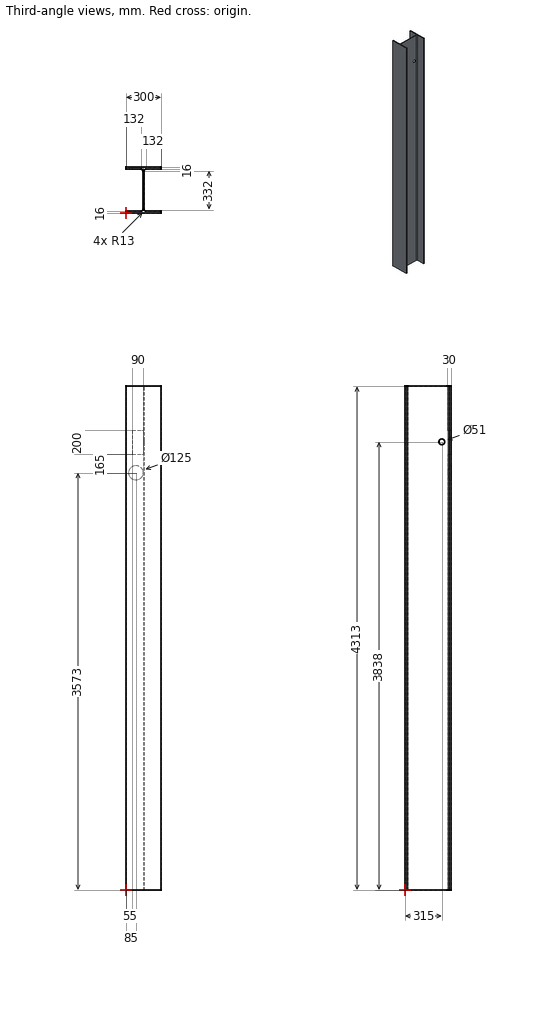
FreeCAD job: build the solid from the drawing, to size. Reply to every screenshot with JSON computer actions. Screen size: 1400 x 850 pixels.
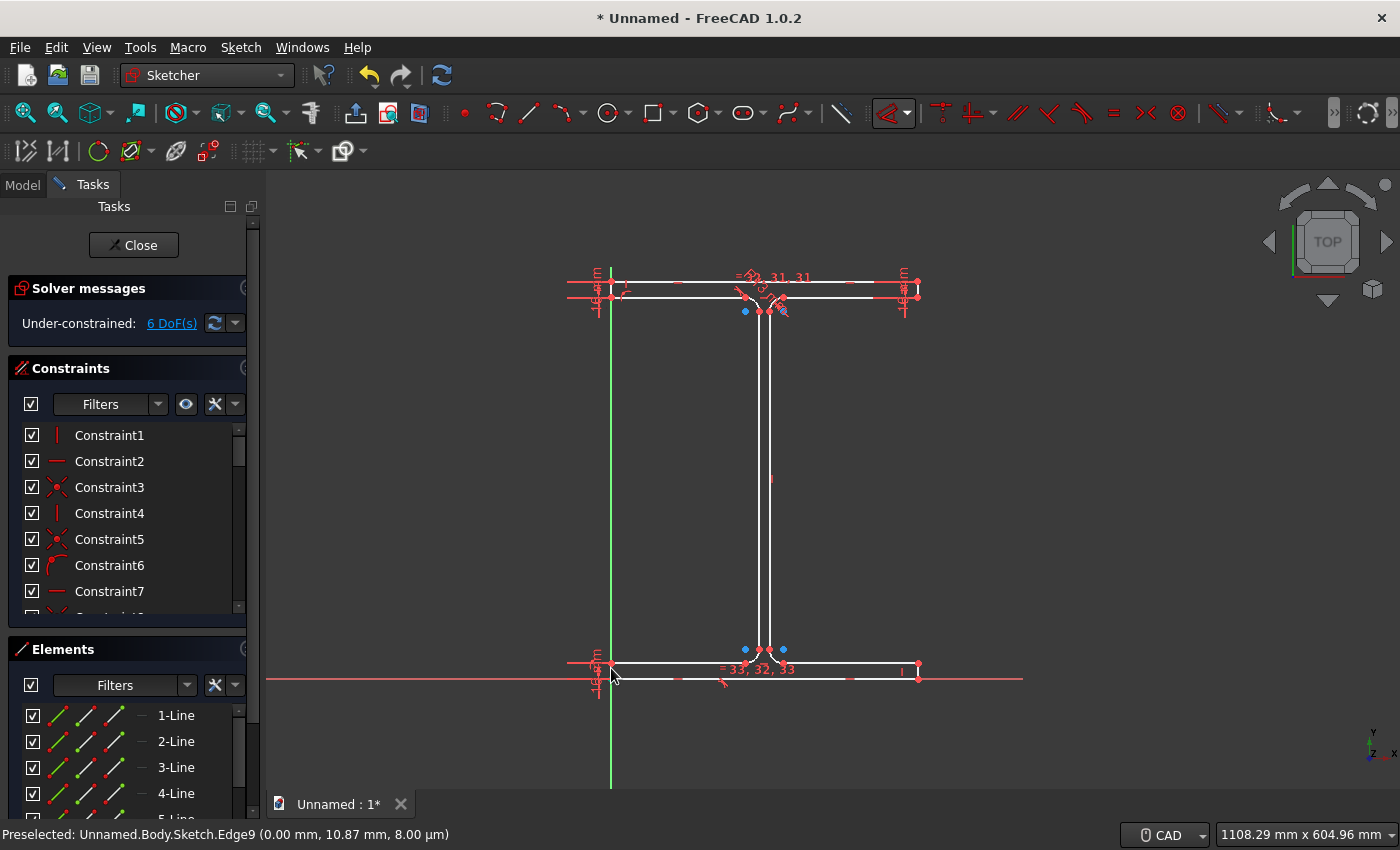
{"action": "scroll", "coordinate": [918, 675], "scroll_direction": "up", "scroll_amount": 6}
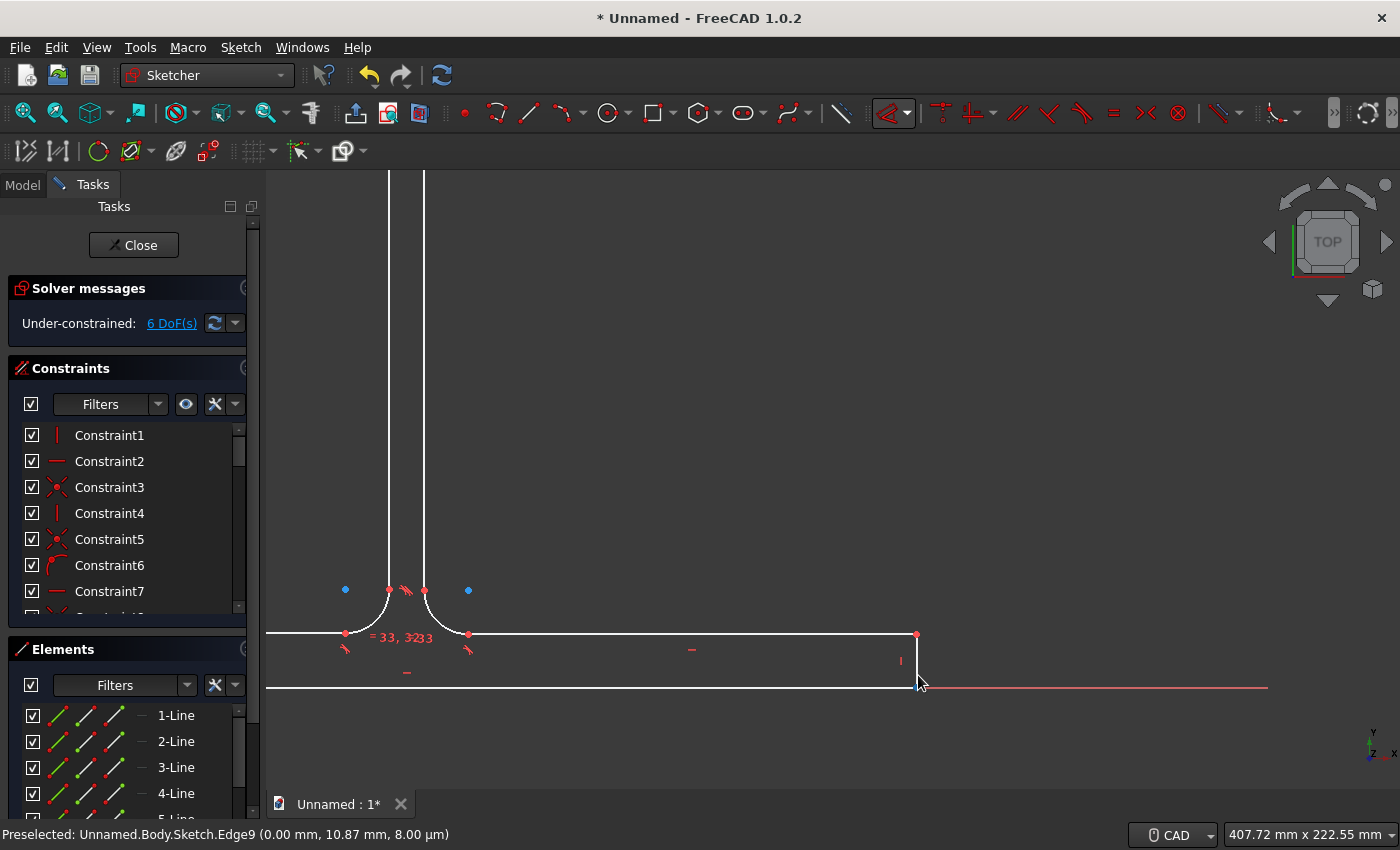
{"action": "left_click", "coordinate": [917, 672]}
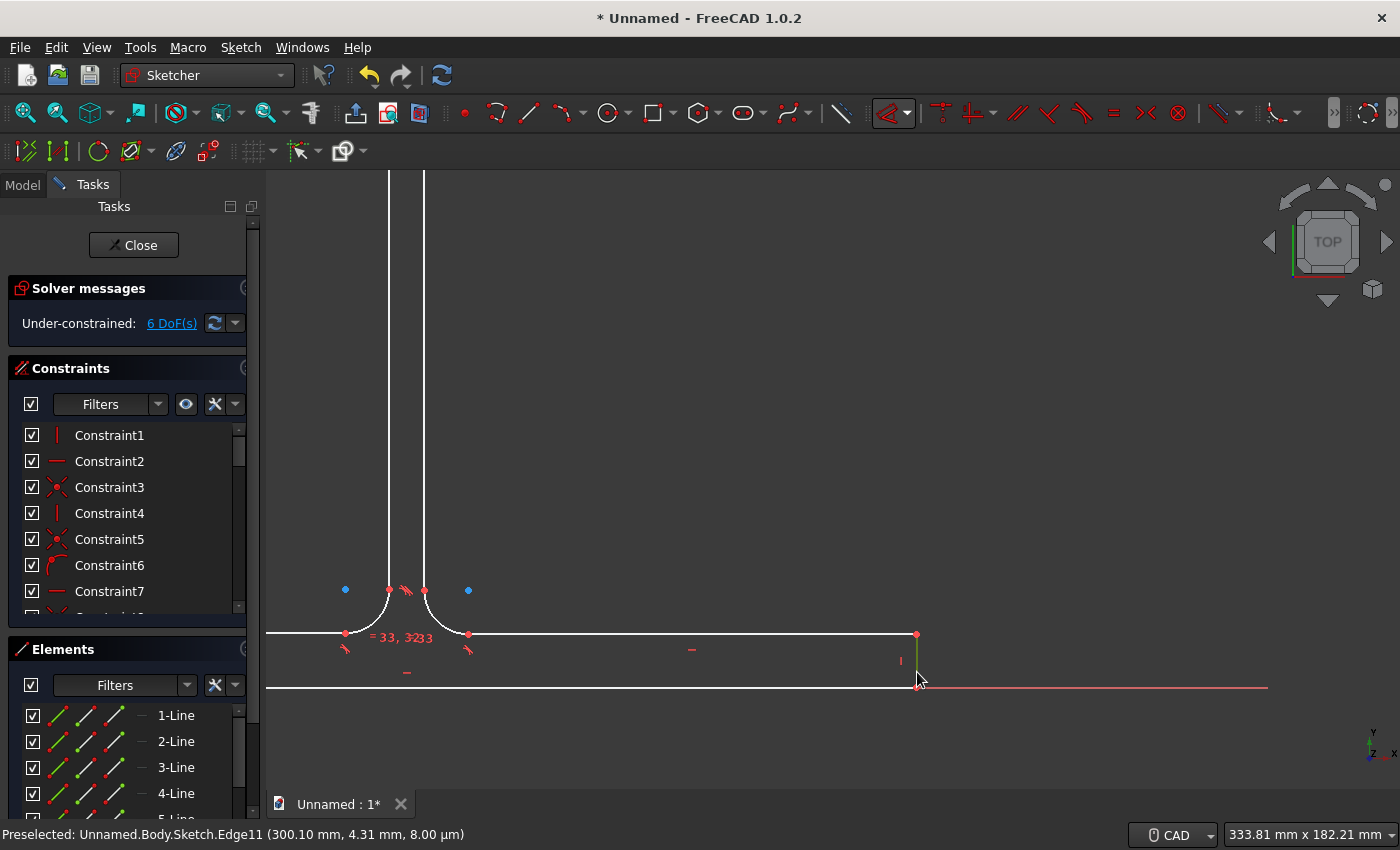
{"action": "key", "text": "i"}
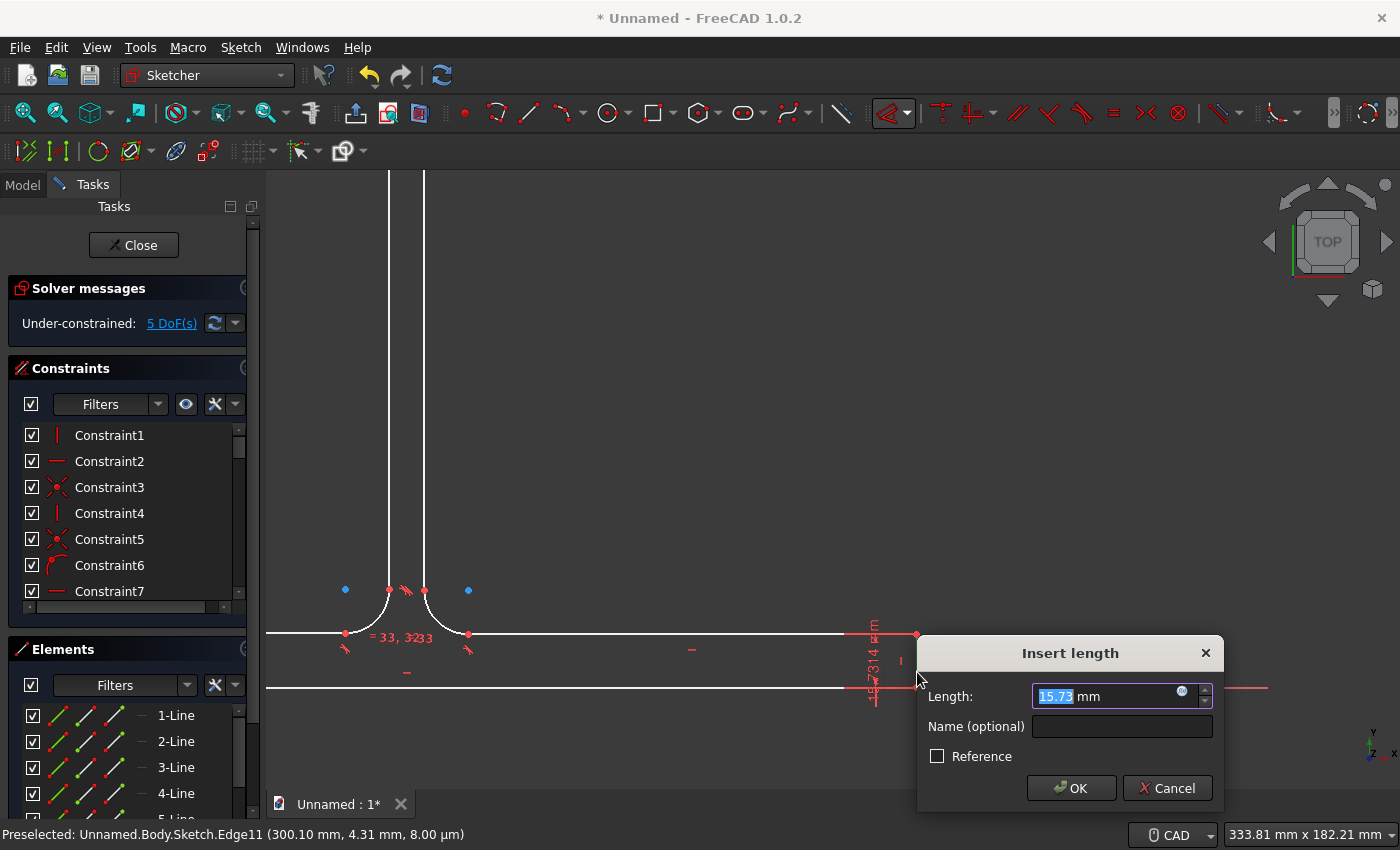
{"action": "type", "text": "16"}
{"action": "key", "text": "Return"}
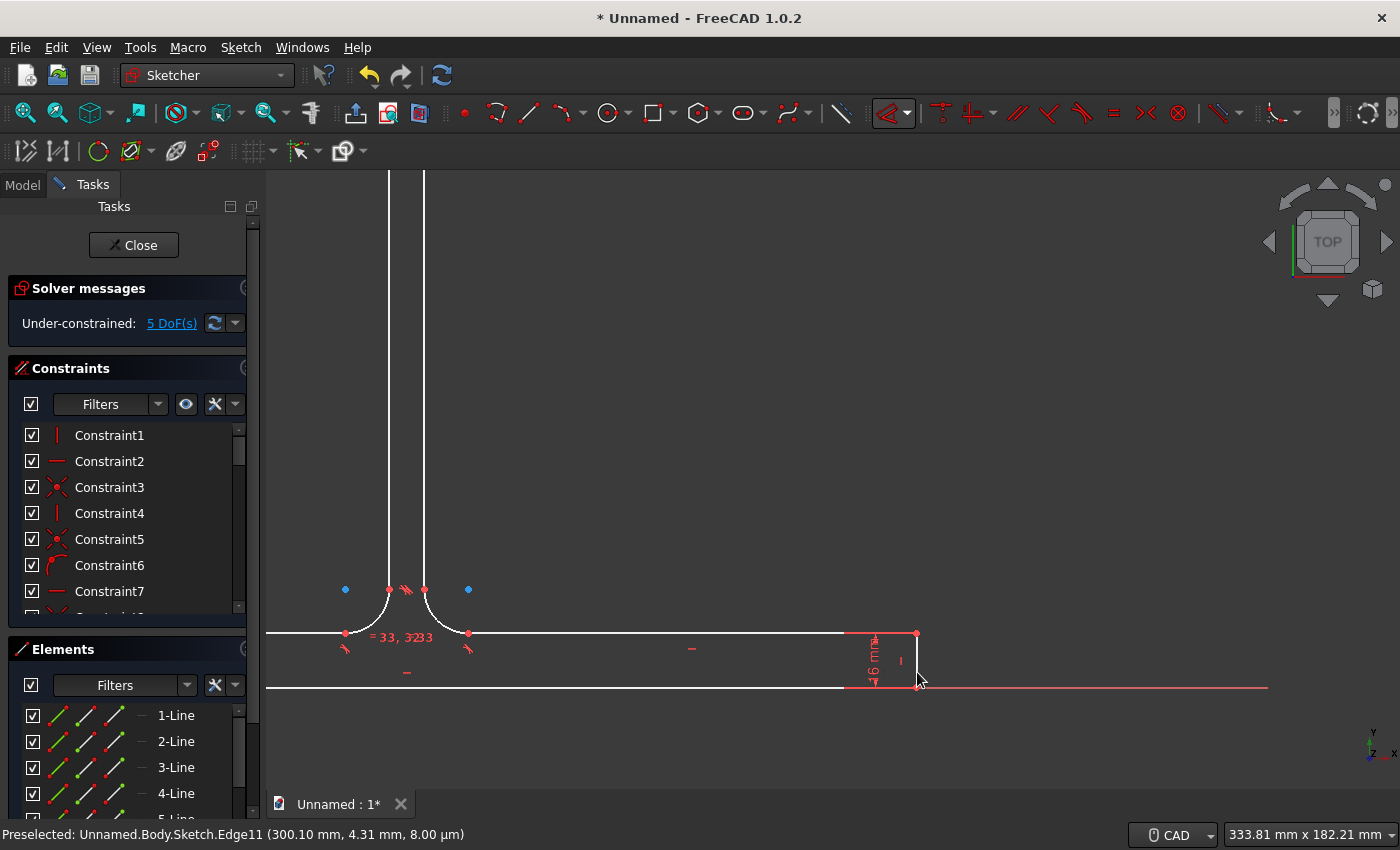
{"action": "left_click", "coordinate": [424, 252]}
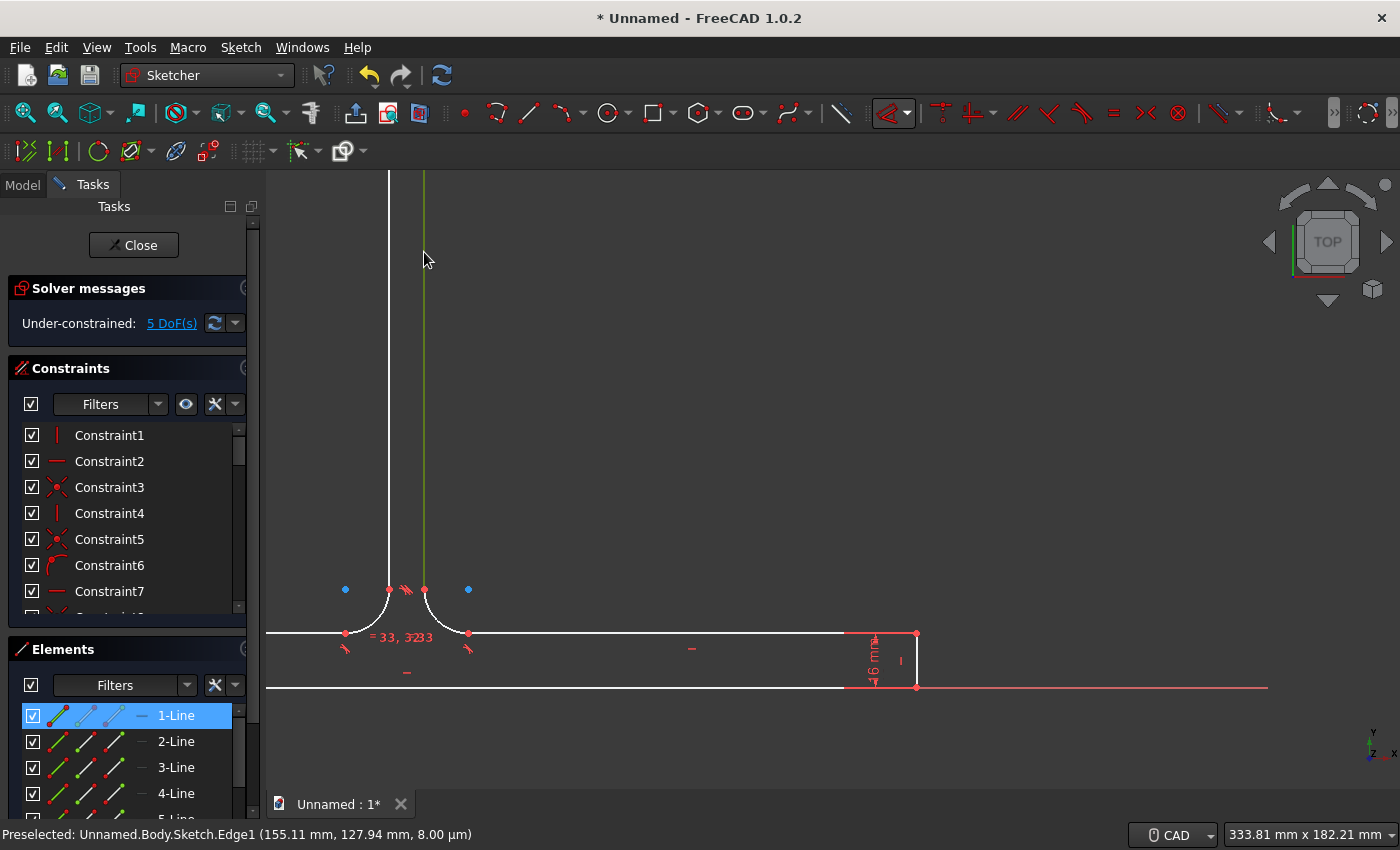
{"action": "key", "text": "i"}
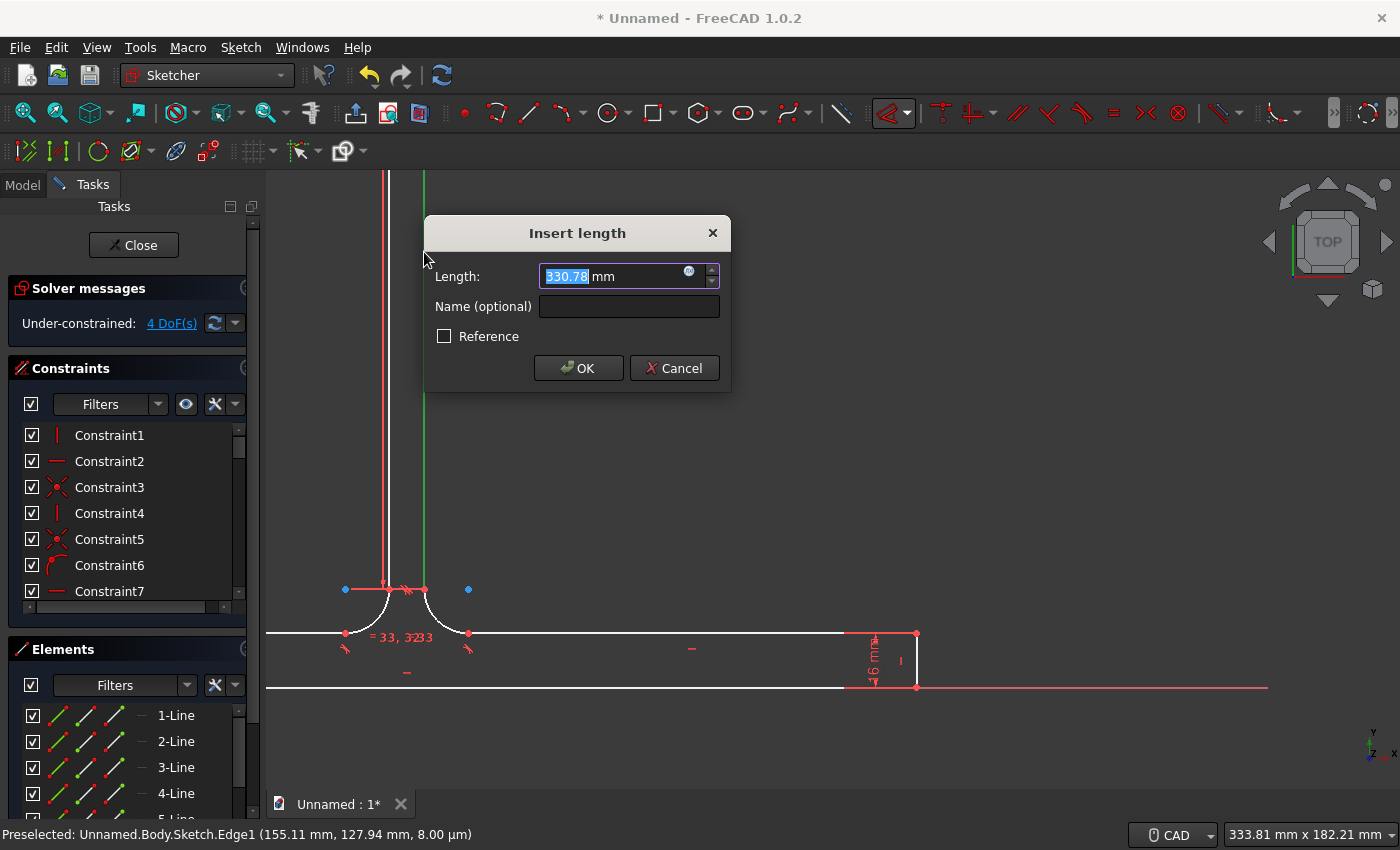
{"action": "type", "text": "332"}
{"action": "key", "text": "Return"}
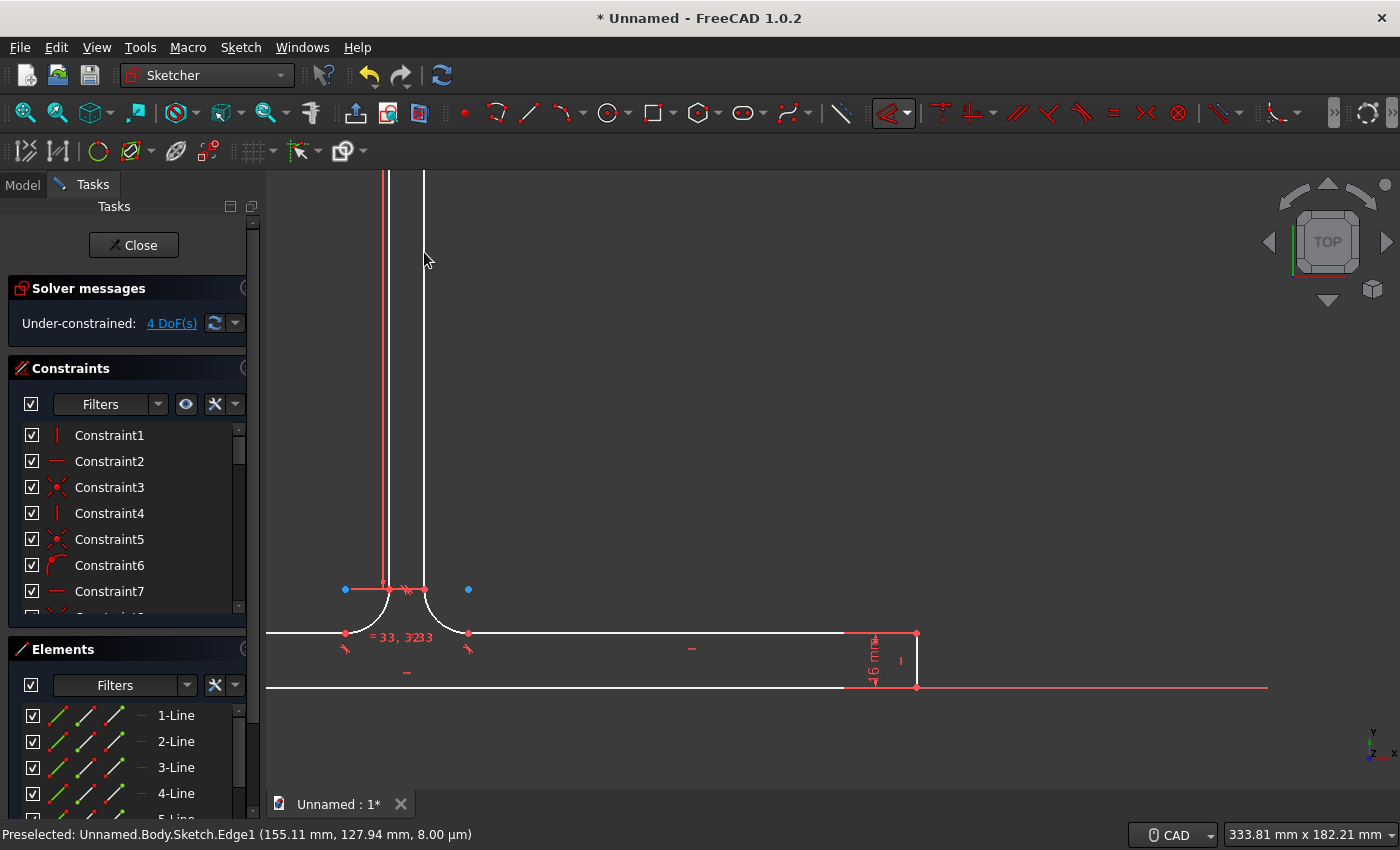
{"action": "scroll", "coordinate": [919, 675], "scroll_direction": "down", "scroll_amount": 6}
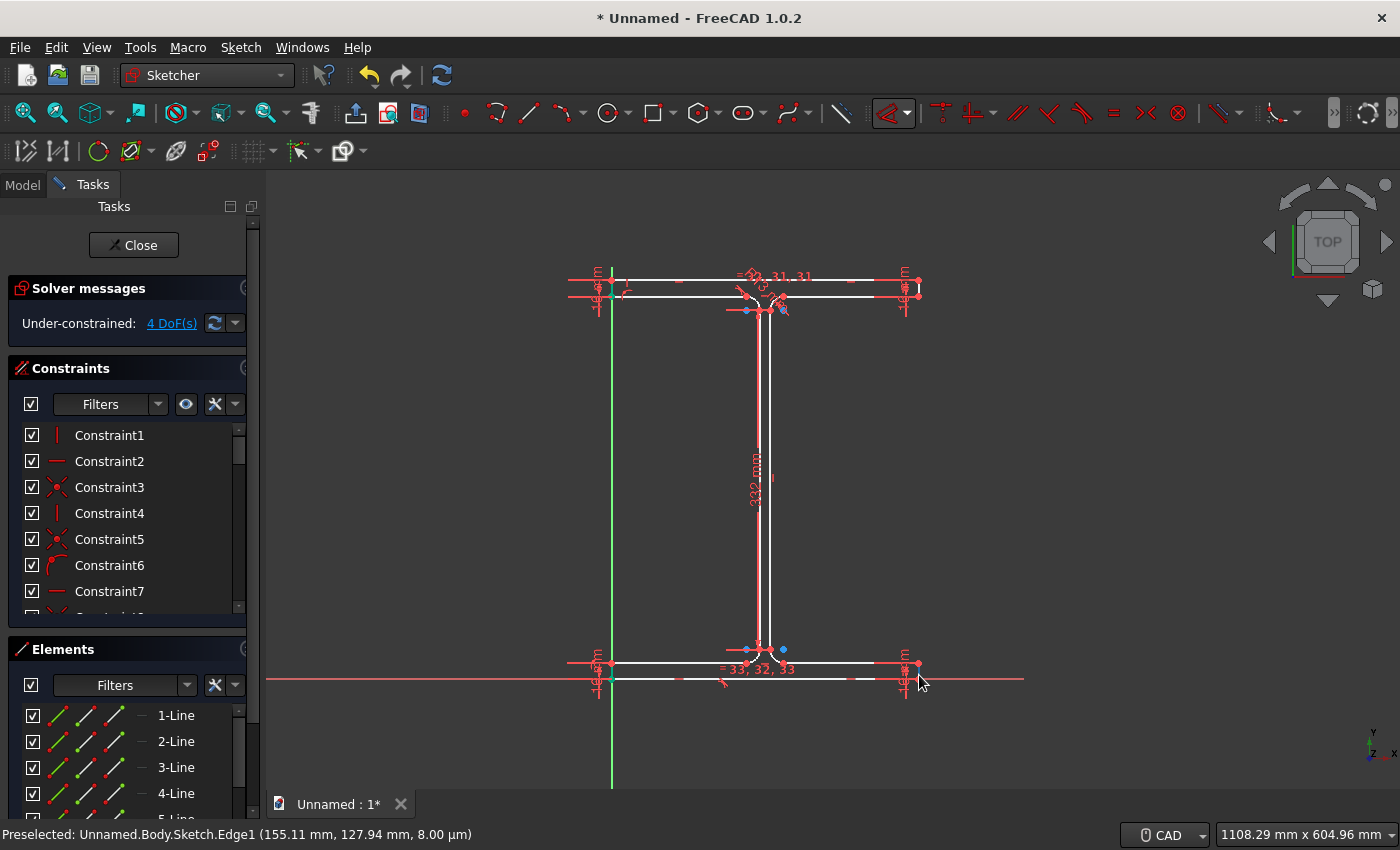
{"action": "left_click", "coordinate": [824, 297]}